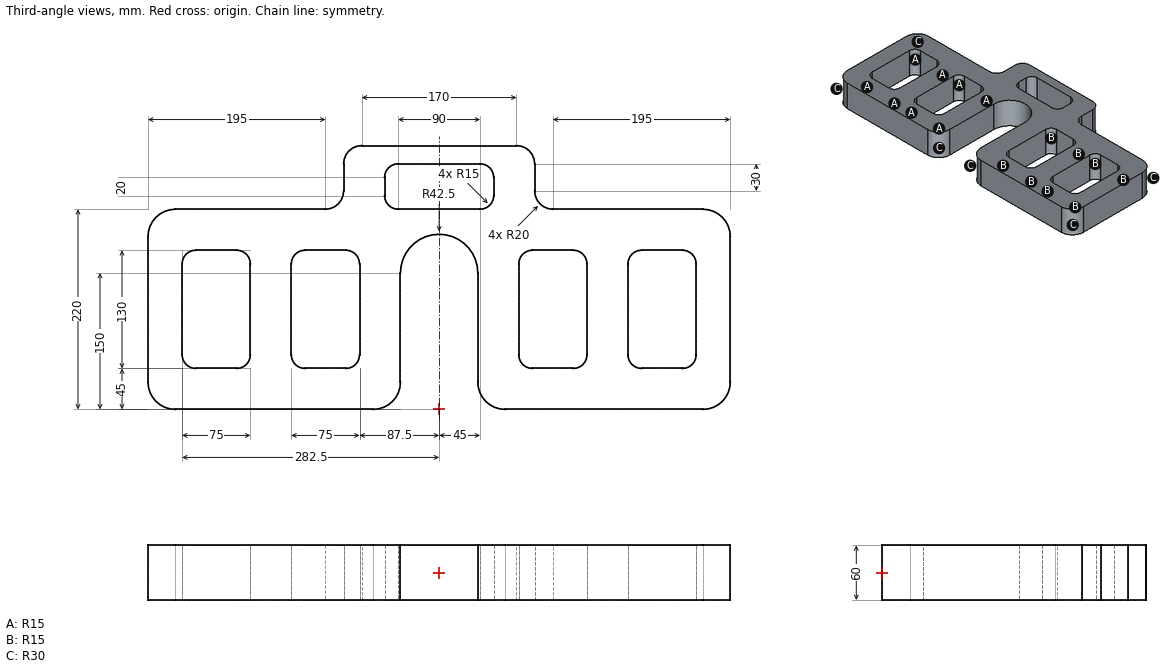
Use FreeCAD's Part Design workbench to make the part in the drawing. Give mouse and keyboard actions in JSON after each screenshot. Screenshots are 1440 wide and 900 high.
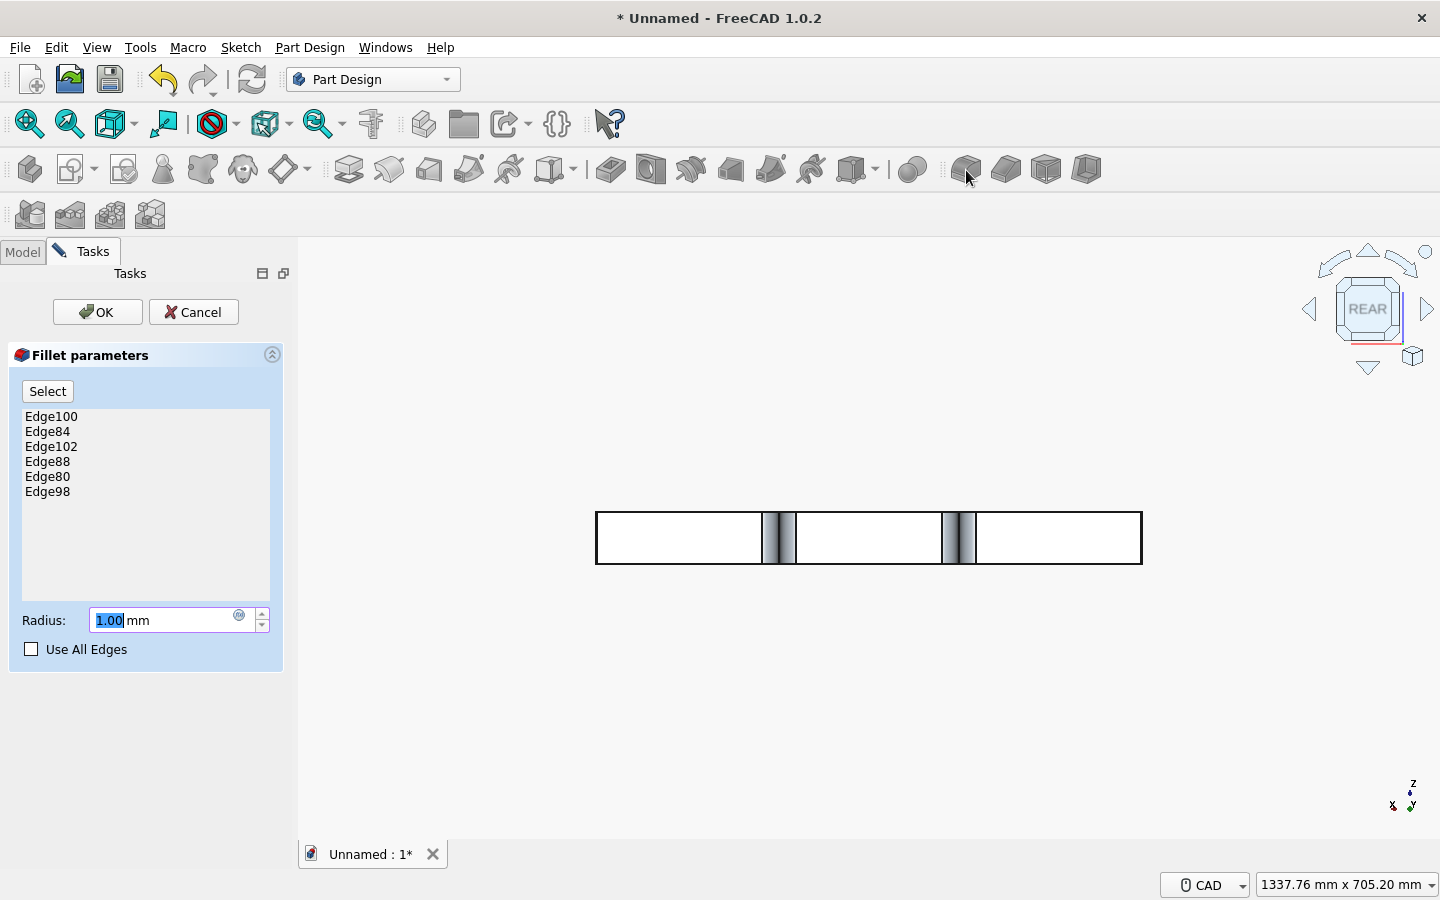
{"action": "type", "text": "30"}
{"action": "key", "text": "Tab"}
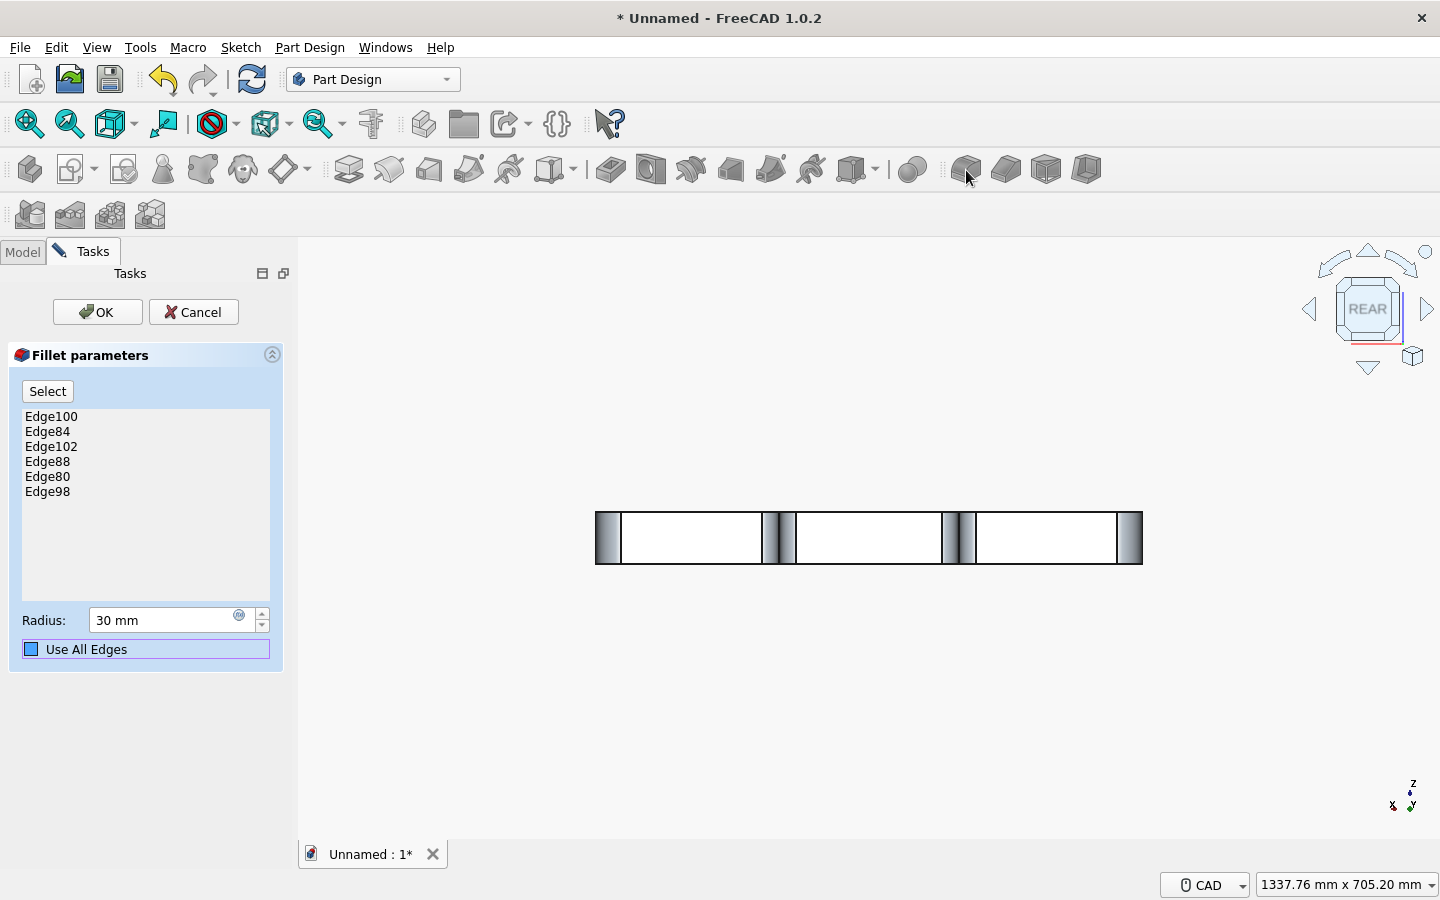
{"action": "left_click", "coordinate": [98, 312]}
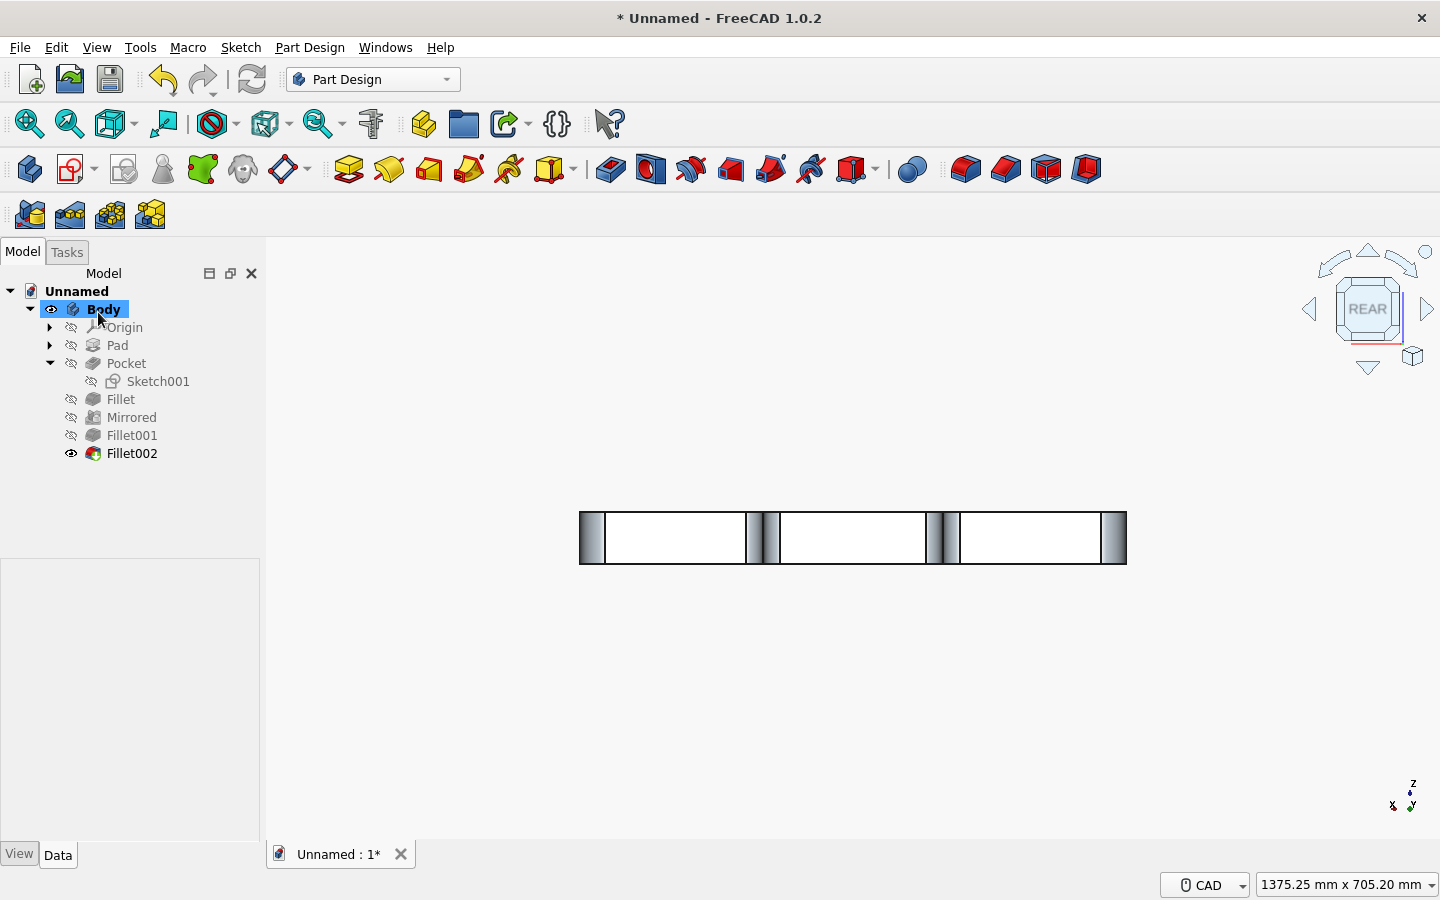
{"action": "key", "text": "0"}